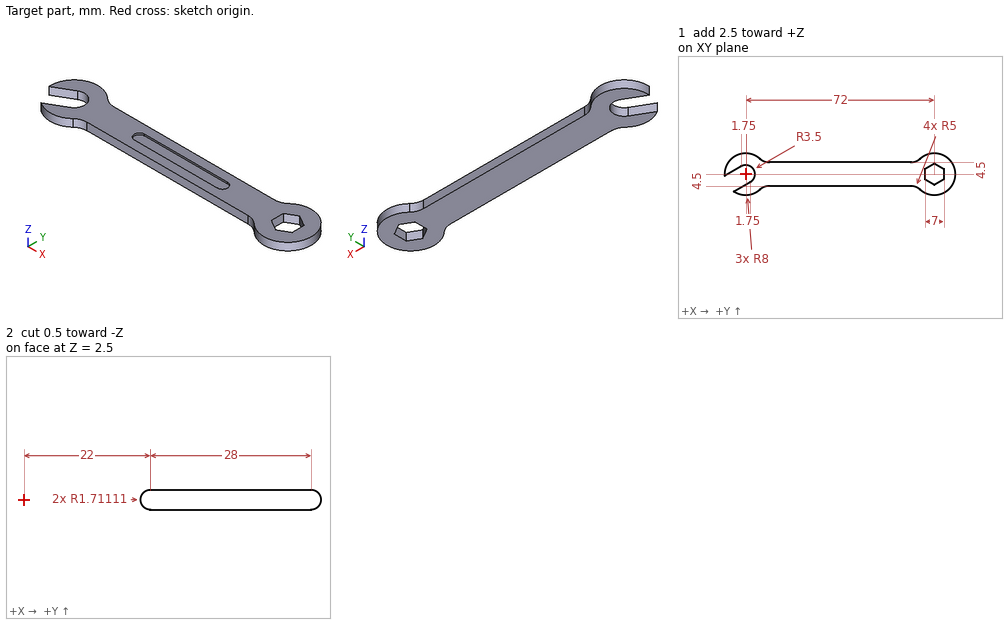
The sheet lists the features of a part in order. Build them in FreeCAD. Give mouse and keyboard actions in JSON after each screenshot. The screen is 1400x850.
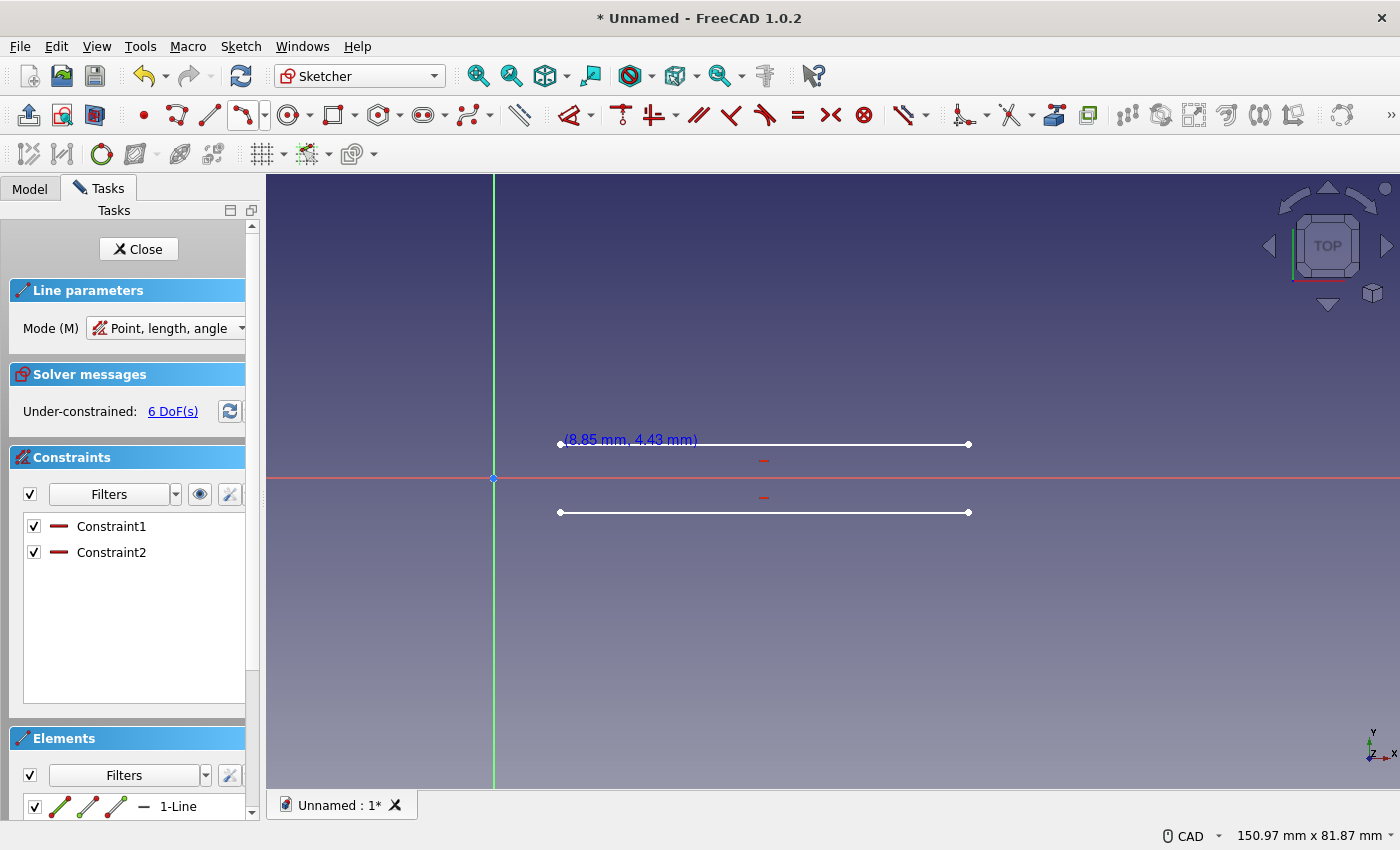
{"action": "scroll", "coordinate": [434, 483], "scroll_direction": "up", "scroll_amount": 7}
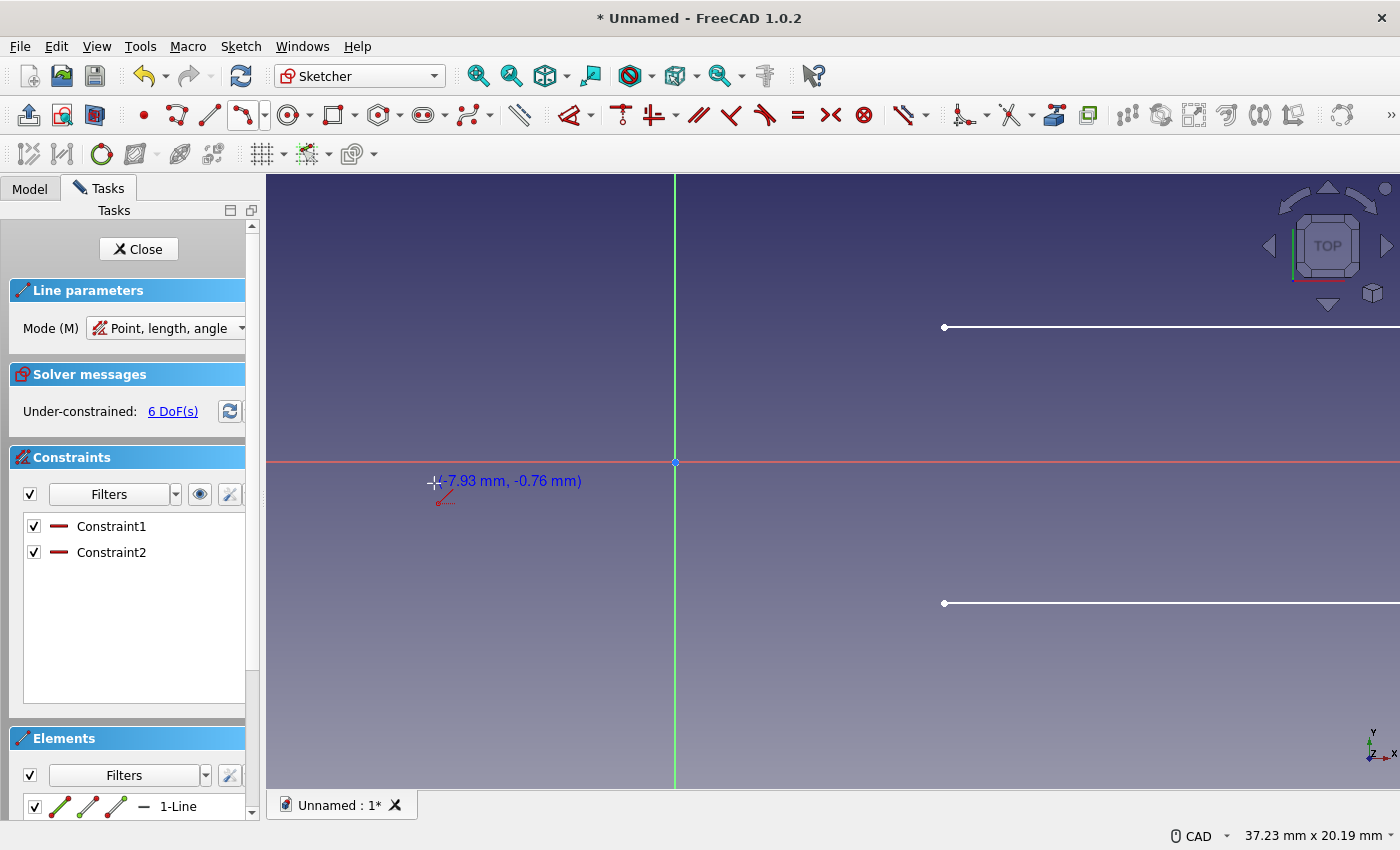
{"action": "left_click", "coordinate": [432, 480]}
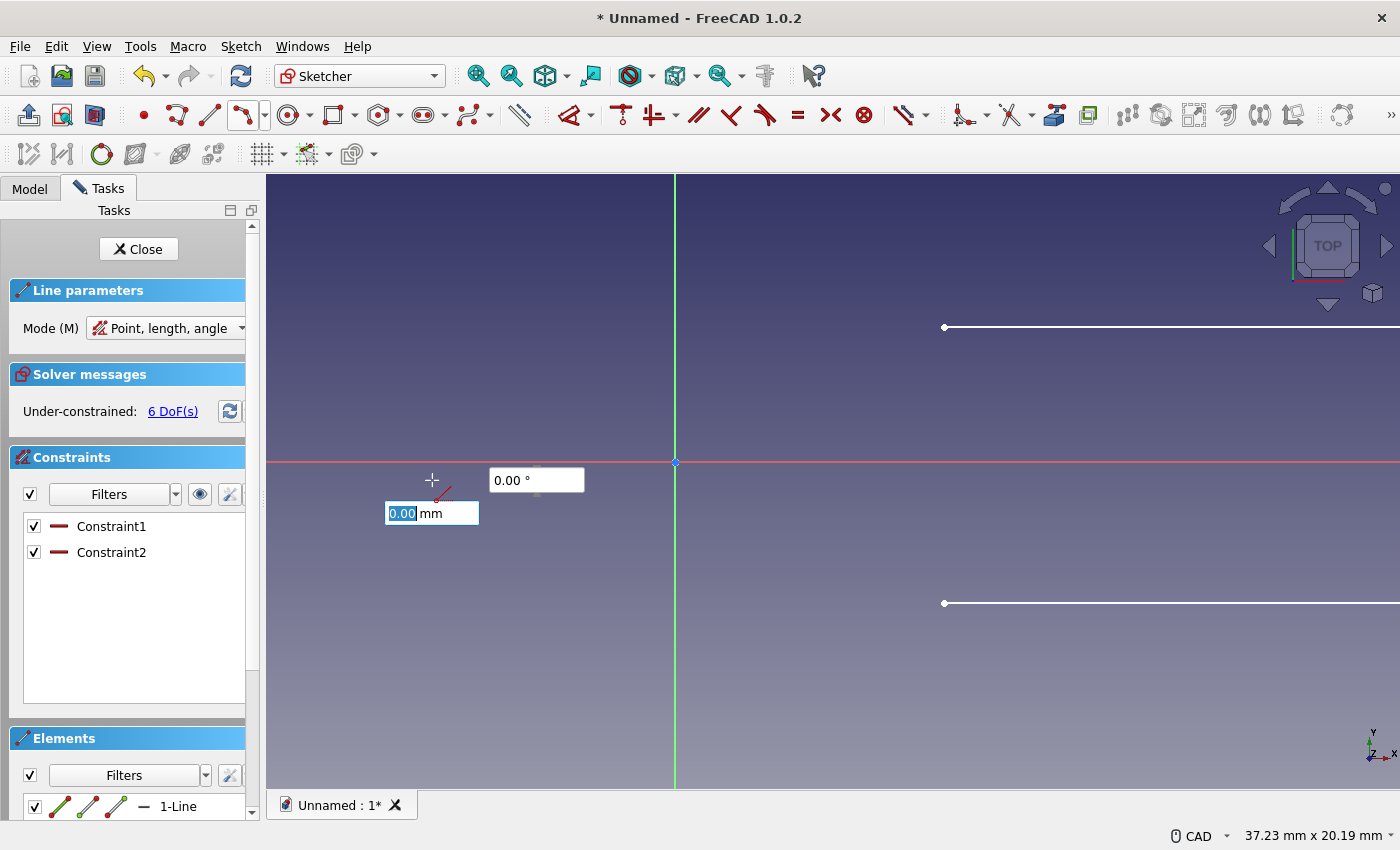
{"action": "scroll", "coordinate": [435, 484], "scroll_direction": "down", "scroll_amount": 7}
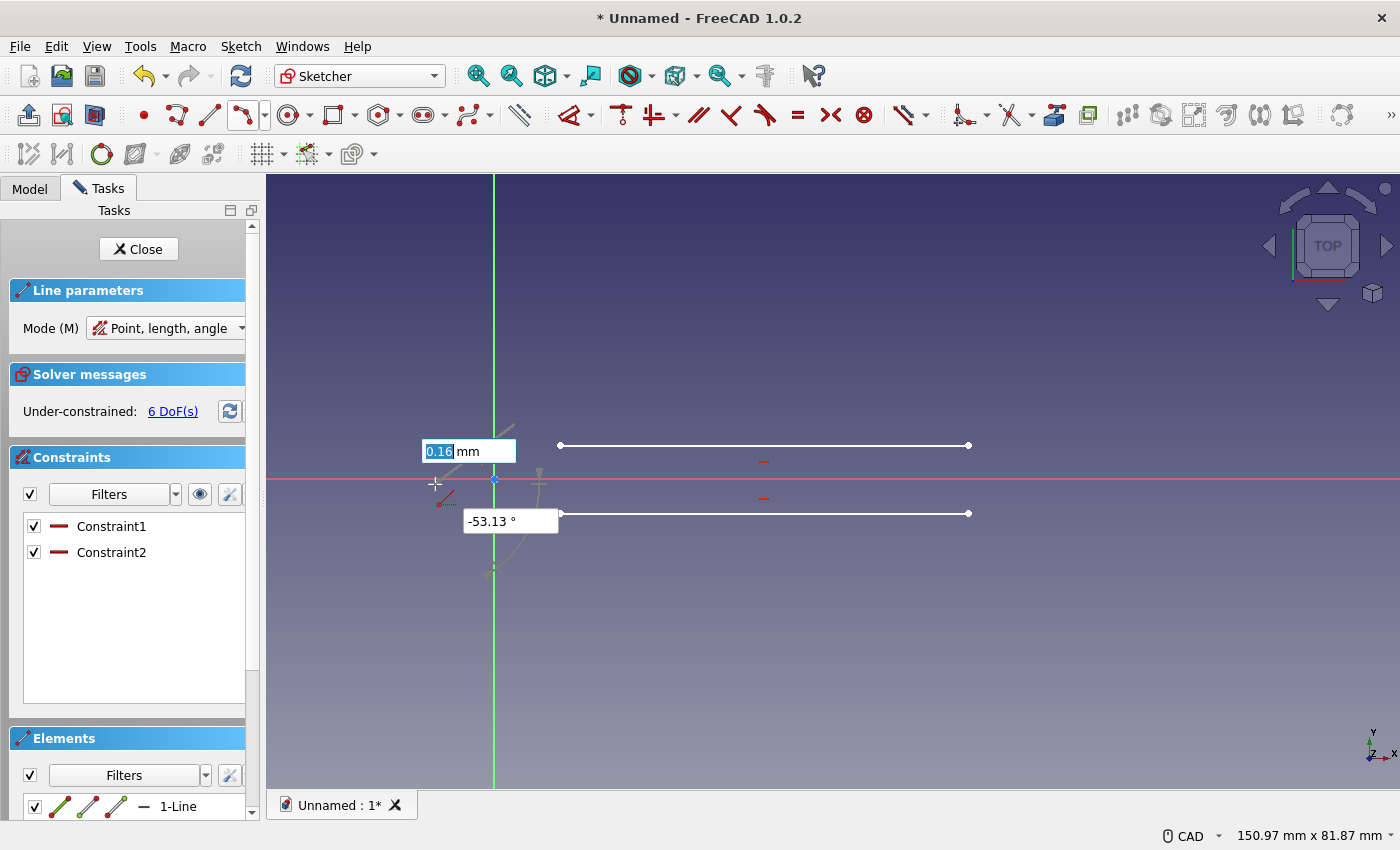
{"action": "left_click", "coordinate": [481, 456]}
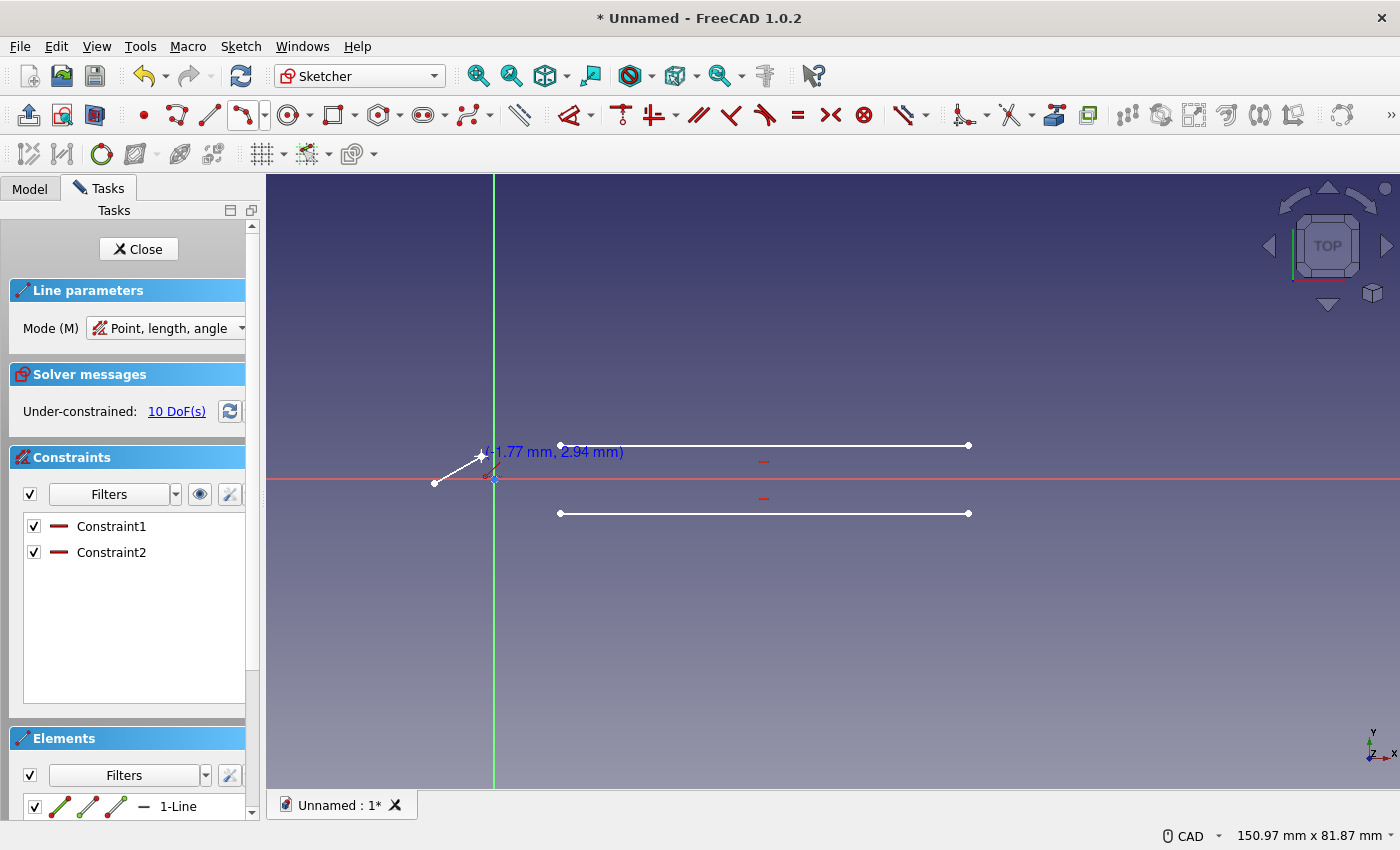
{"action": "left_click", "coordinate": [507, 502]}
{"action": "left_click", "coordinate": [461, 529]}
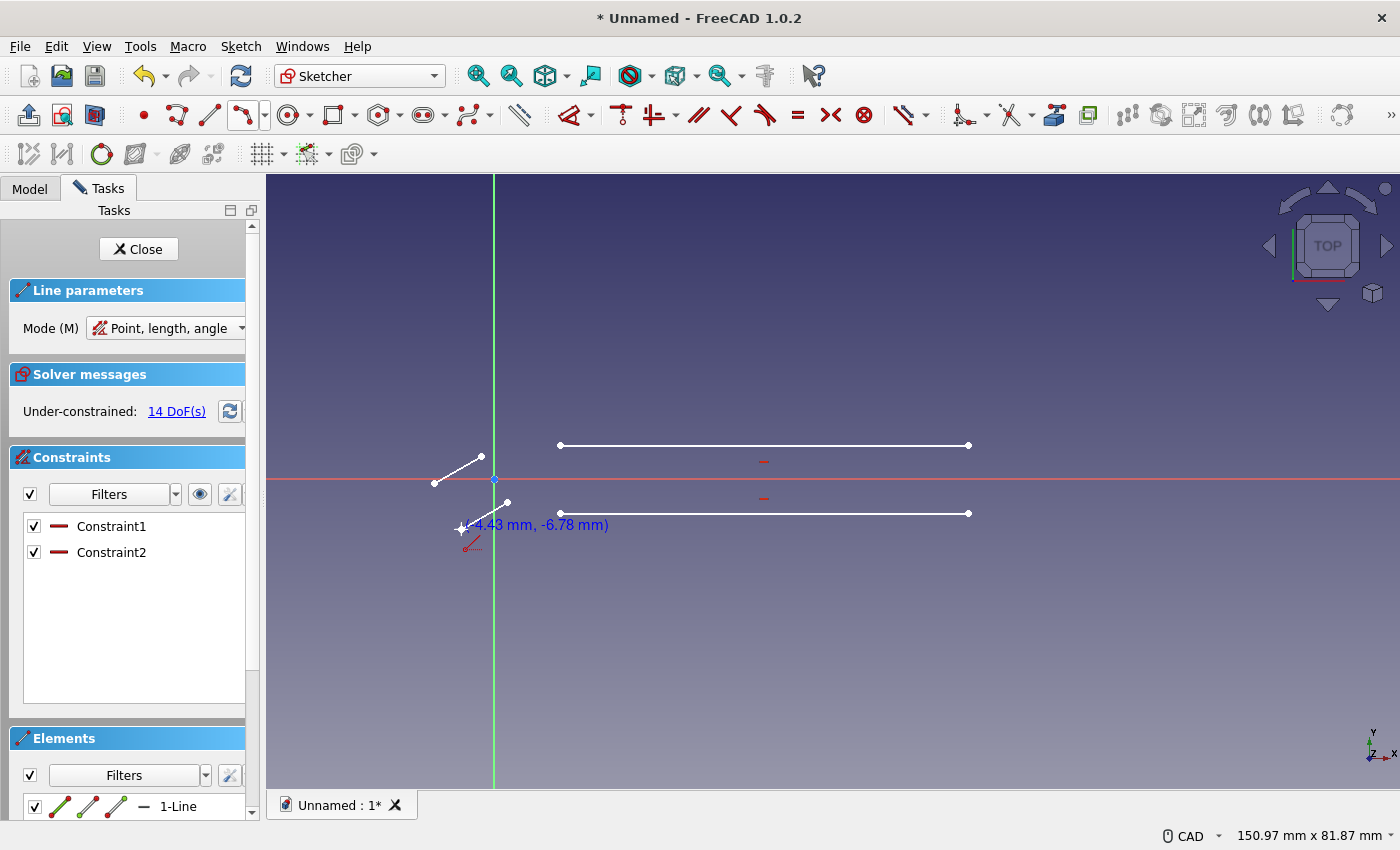
{"action": "key", "text": "g 3 a"}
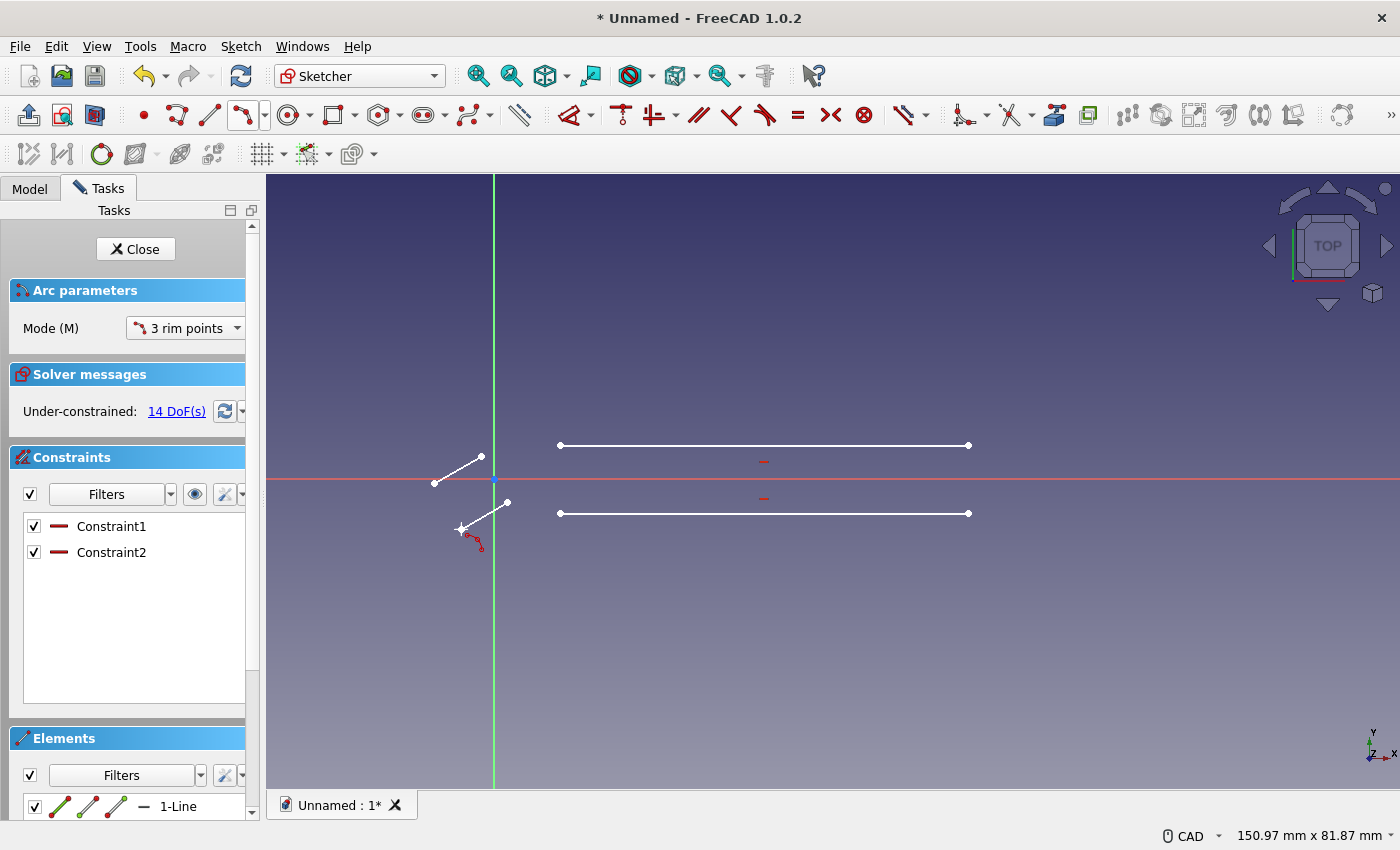
{"action": "left_click", "coordinate": [969, 514]}
{"action": "left_click", "coordinate": [994, 523]}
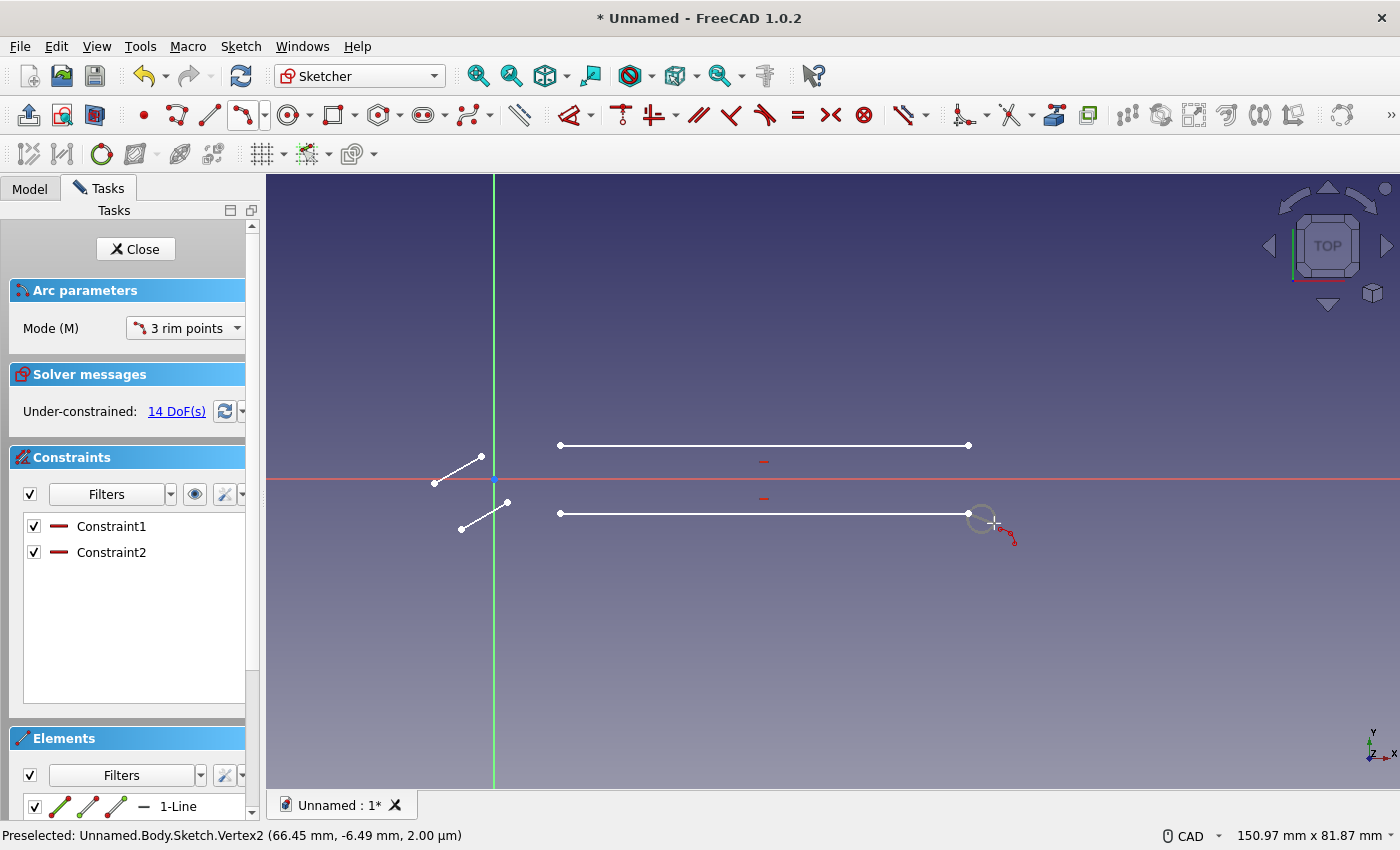
{"action": "scroll", "coordinate": [982, 515], "scroll_direction": "up", "scroll_amount": 10}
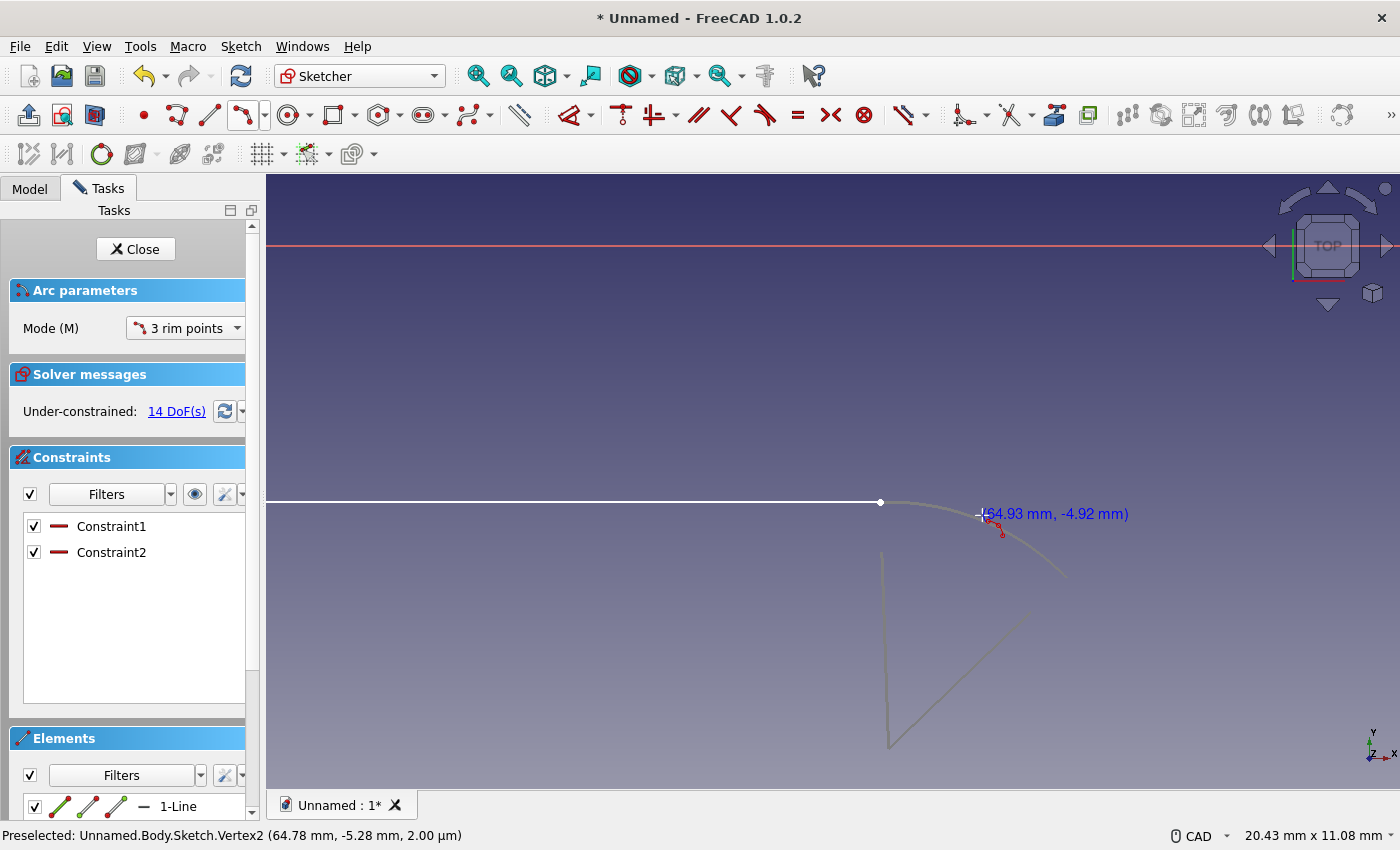
{"action": "left_click", "coordinate": [980, 515]}